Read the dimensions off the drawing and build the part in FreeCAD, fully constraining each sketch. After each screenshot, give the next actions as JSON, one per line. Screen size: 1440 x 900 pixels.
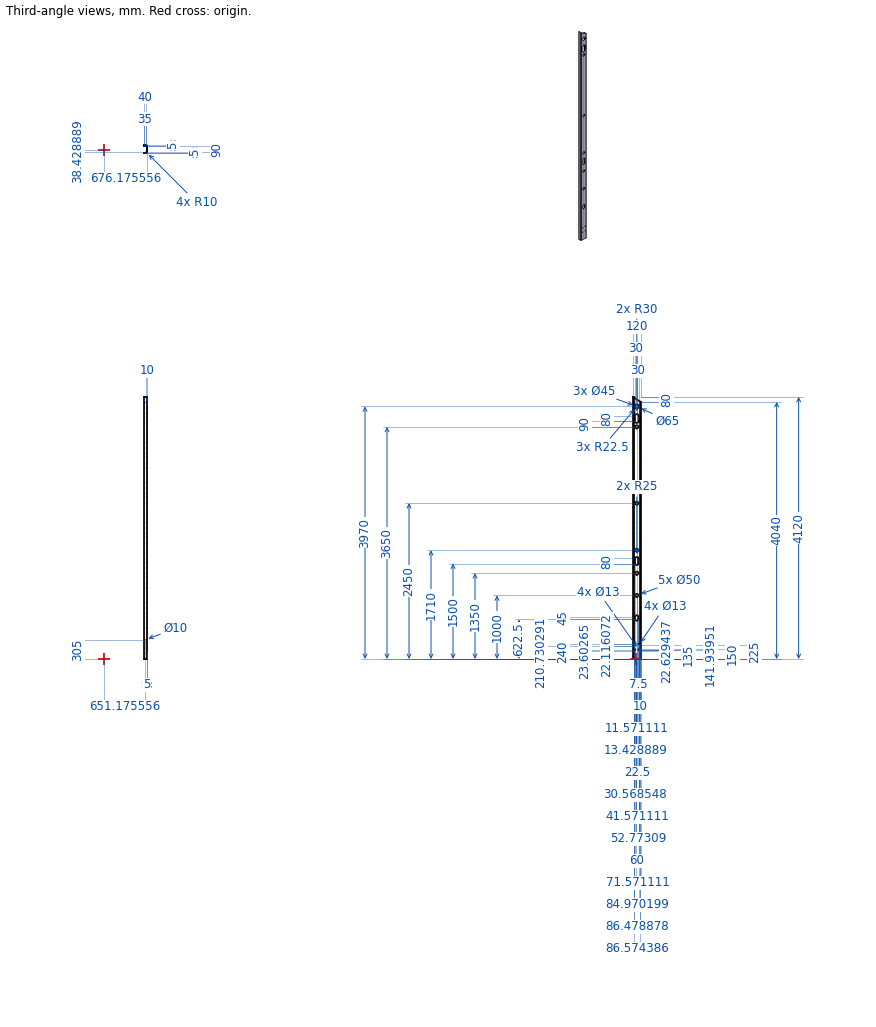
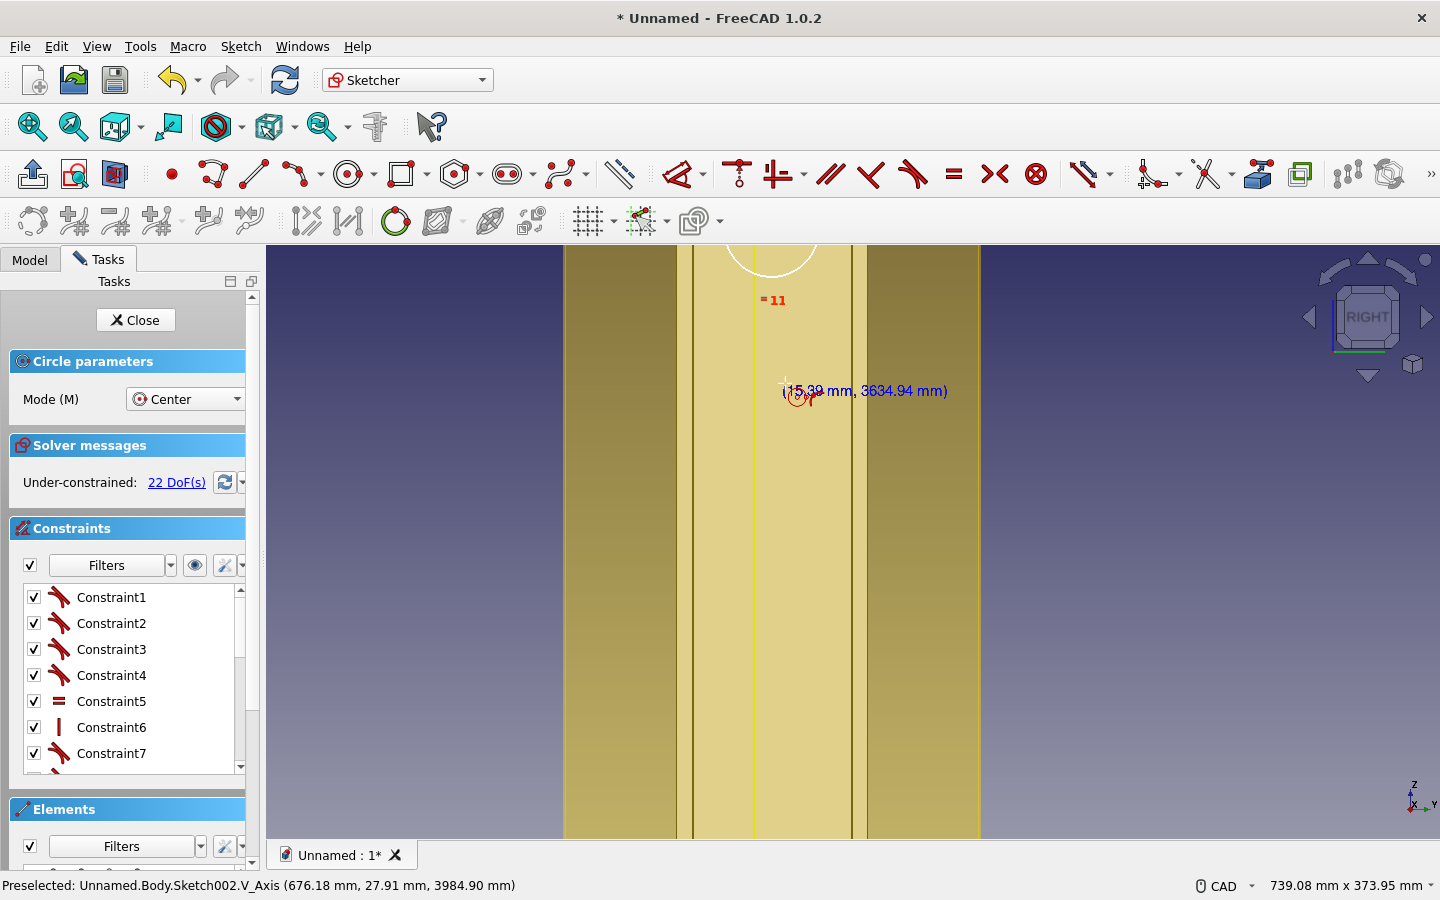
{"action": "left_click", "coordinate": [772, 372]}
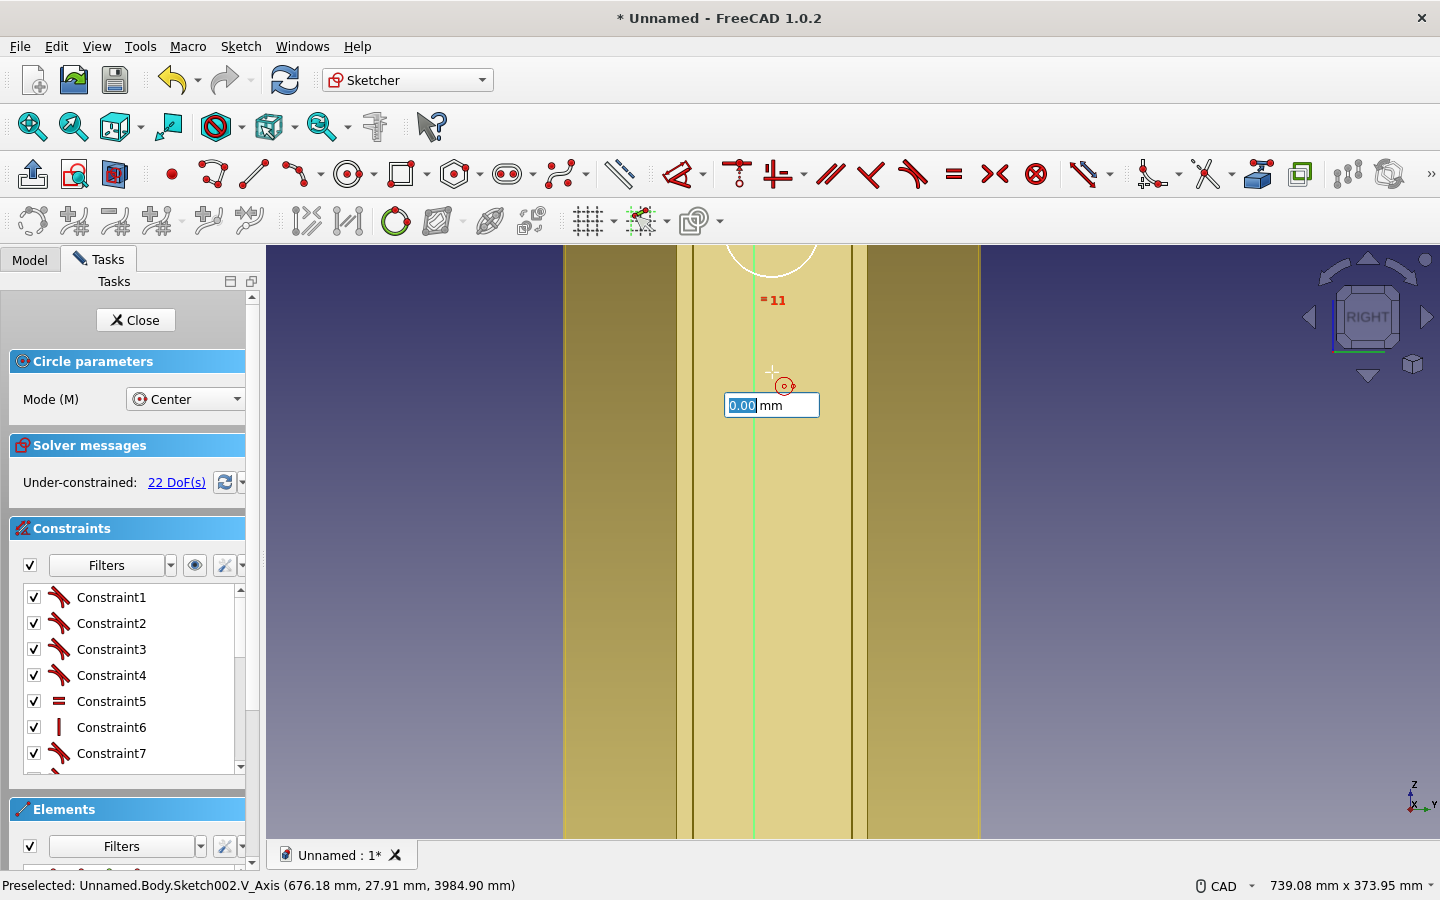
{"action": "scroll", "coordinate": [785, 383], "scroll_direction": "down", "scroll_amount": 14}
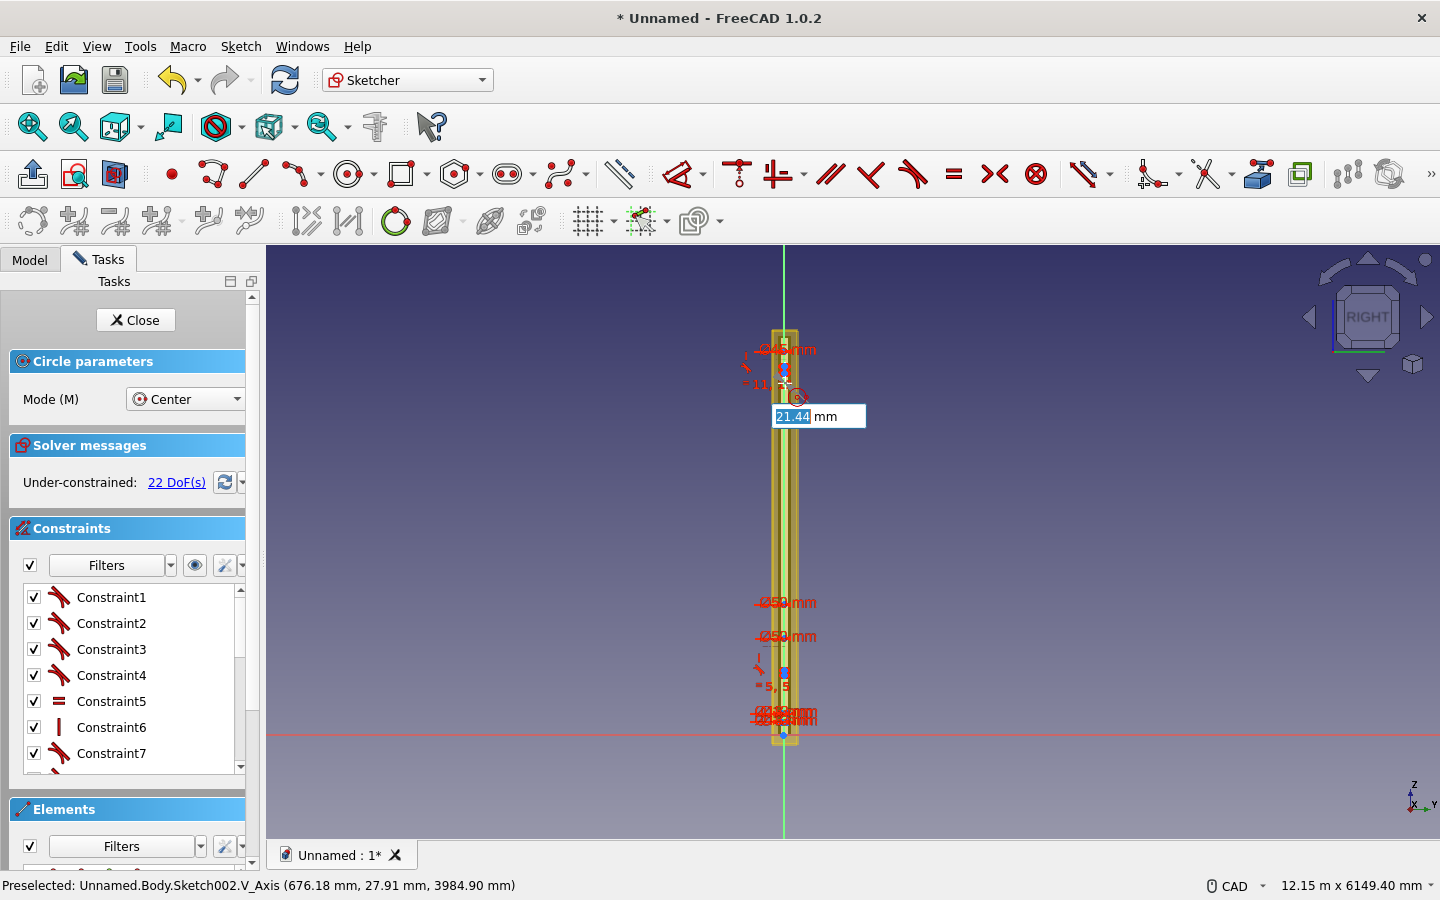
{"action": "scroll", "coordinate": [786, 381], "scroll_direction": "up", "scroll_amount": 9}
{"action": "mouse_move", "coordinate": [786, 379]}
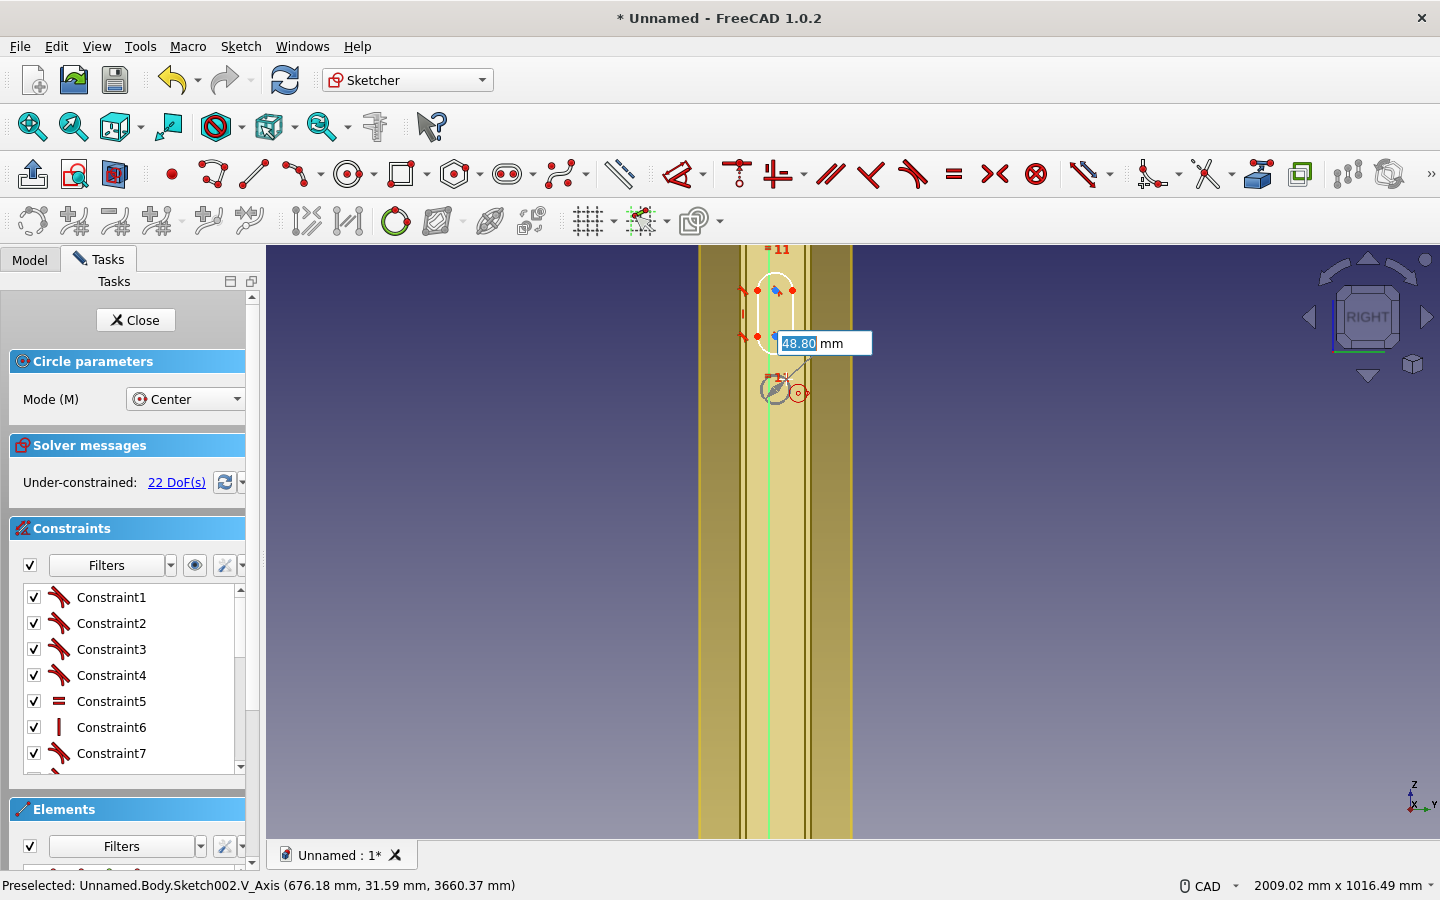
{"action": "type", "text": "50"}
{"action": "key", "text": "Return"}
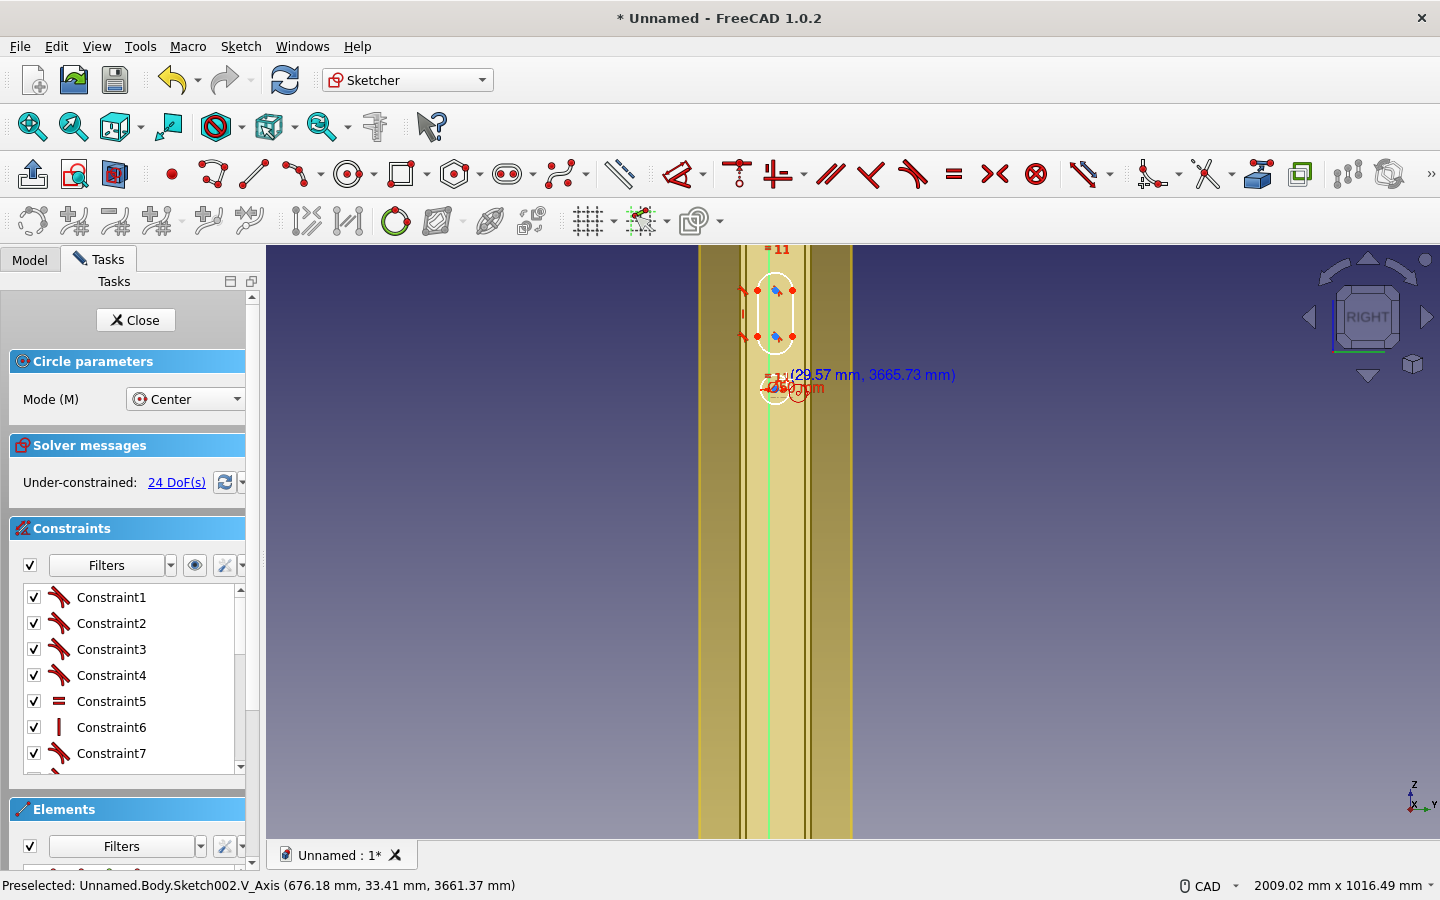
{"action": "scroll", "coordinate": [786, 381], "scroll_direction": "down", "scroll_amount": 9}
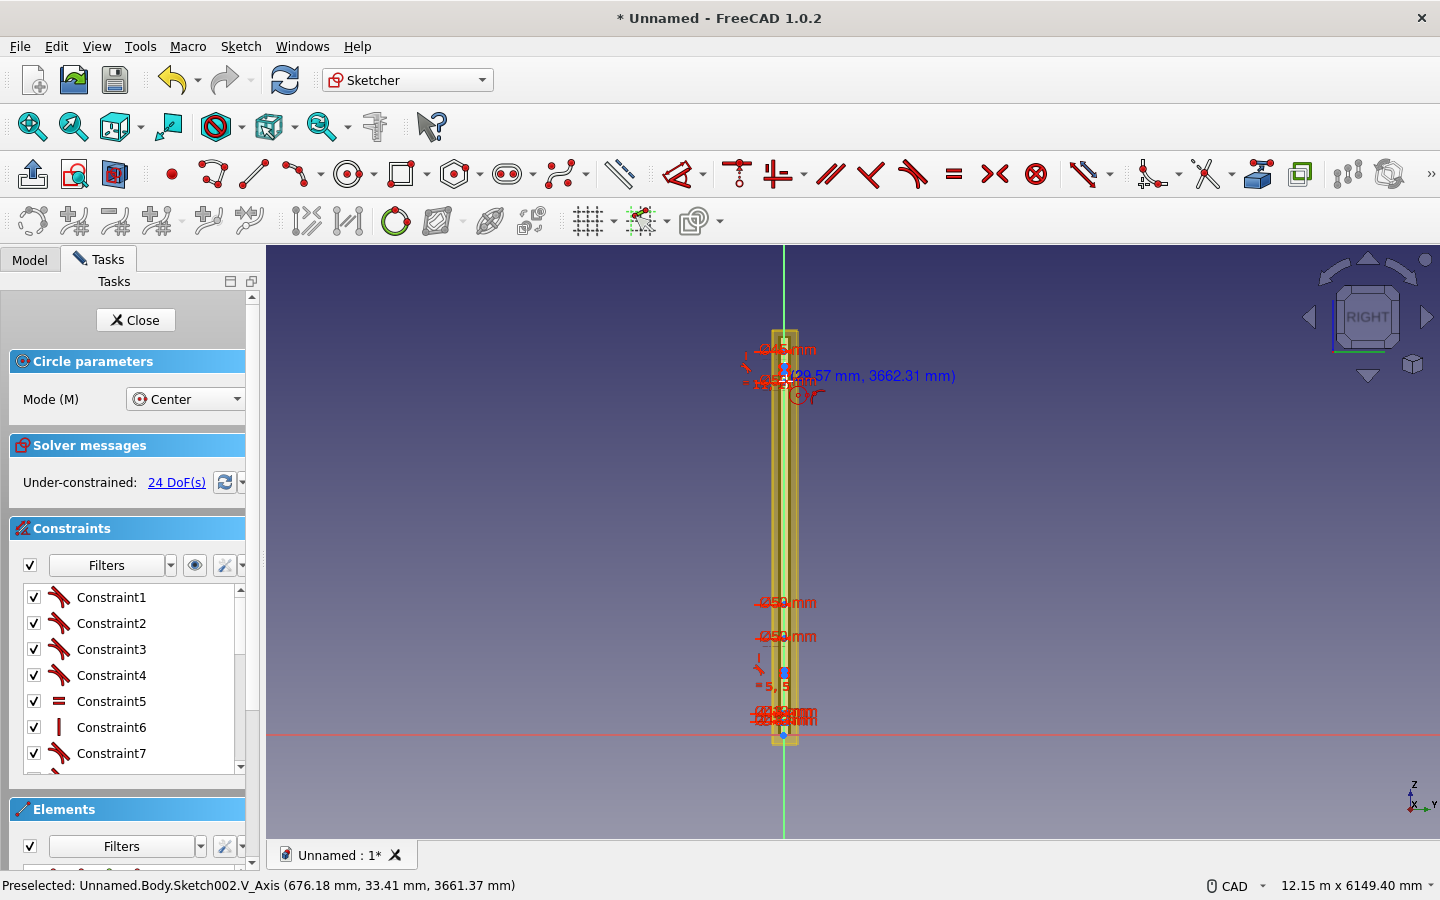
{"action": "scroll", "coordinate": [785, 570], "scroll_direction": "up", "scroll_amount": 14}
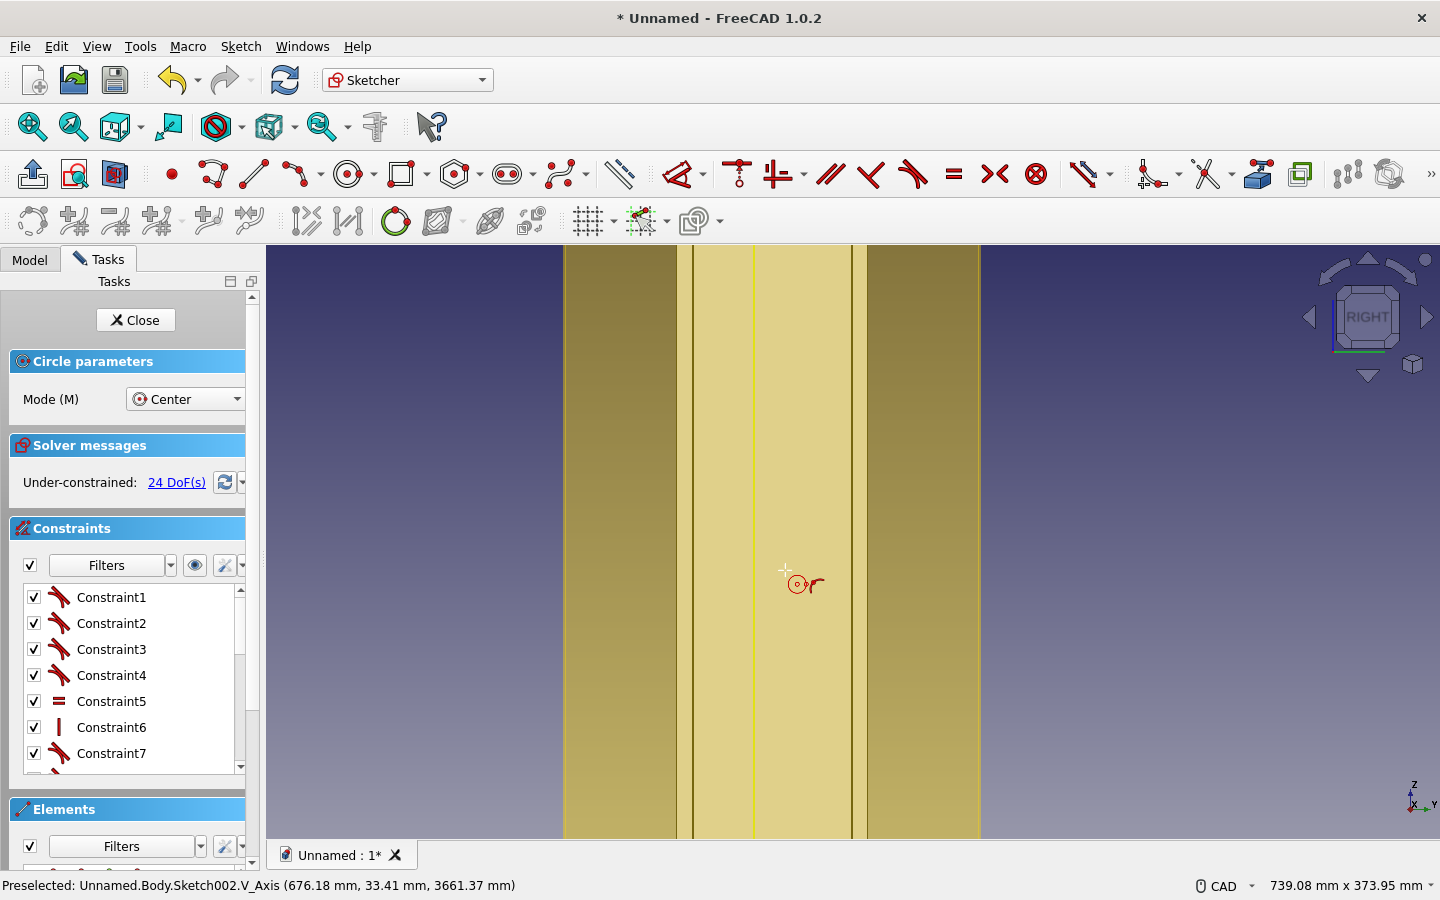
{"action": "left_click", "coordinate": [772, 561]}